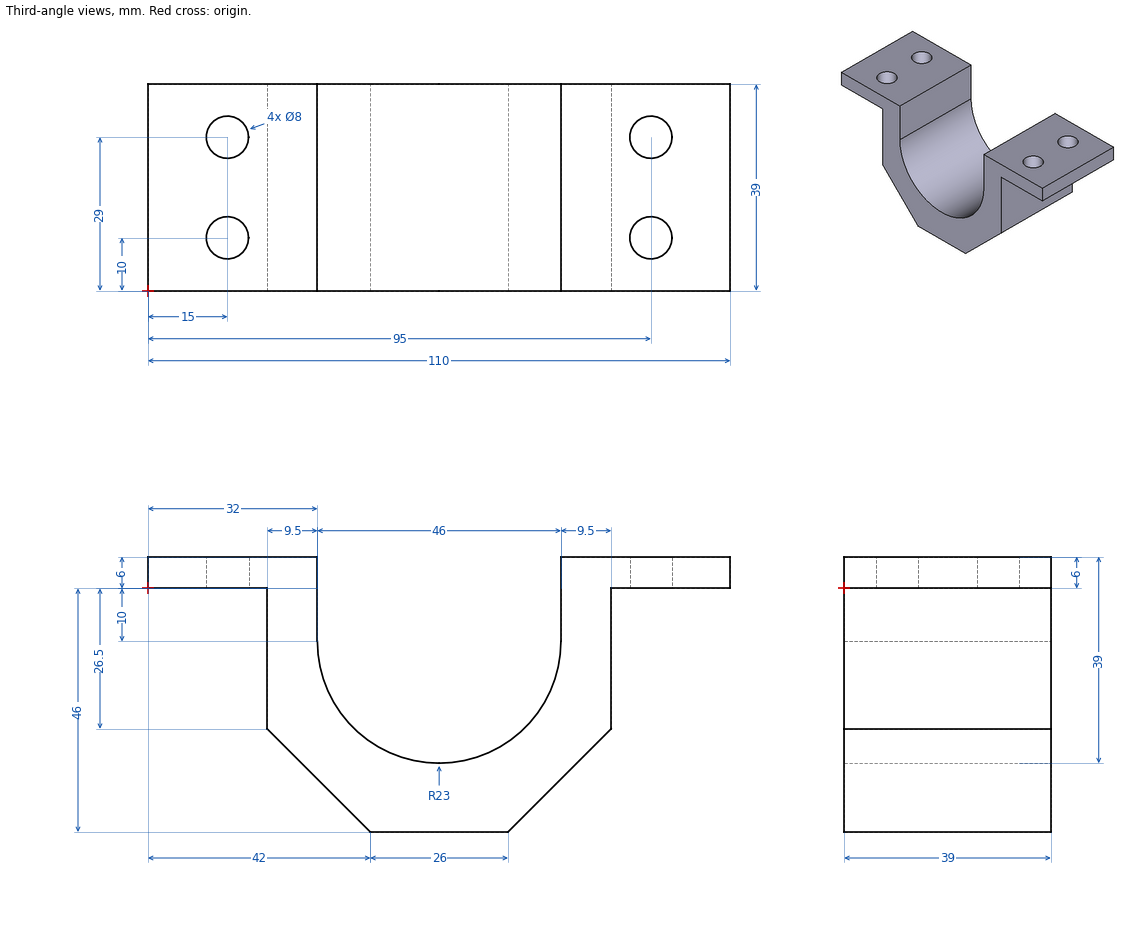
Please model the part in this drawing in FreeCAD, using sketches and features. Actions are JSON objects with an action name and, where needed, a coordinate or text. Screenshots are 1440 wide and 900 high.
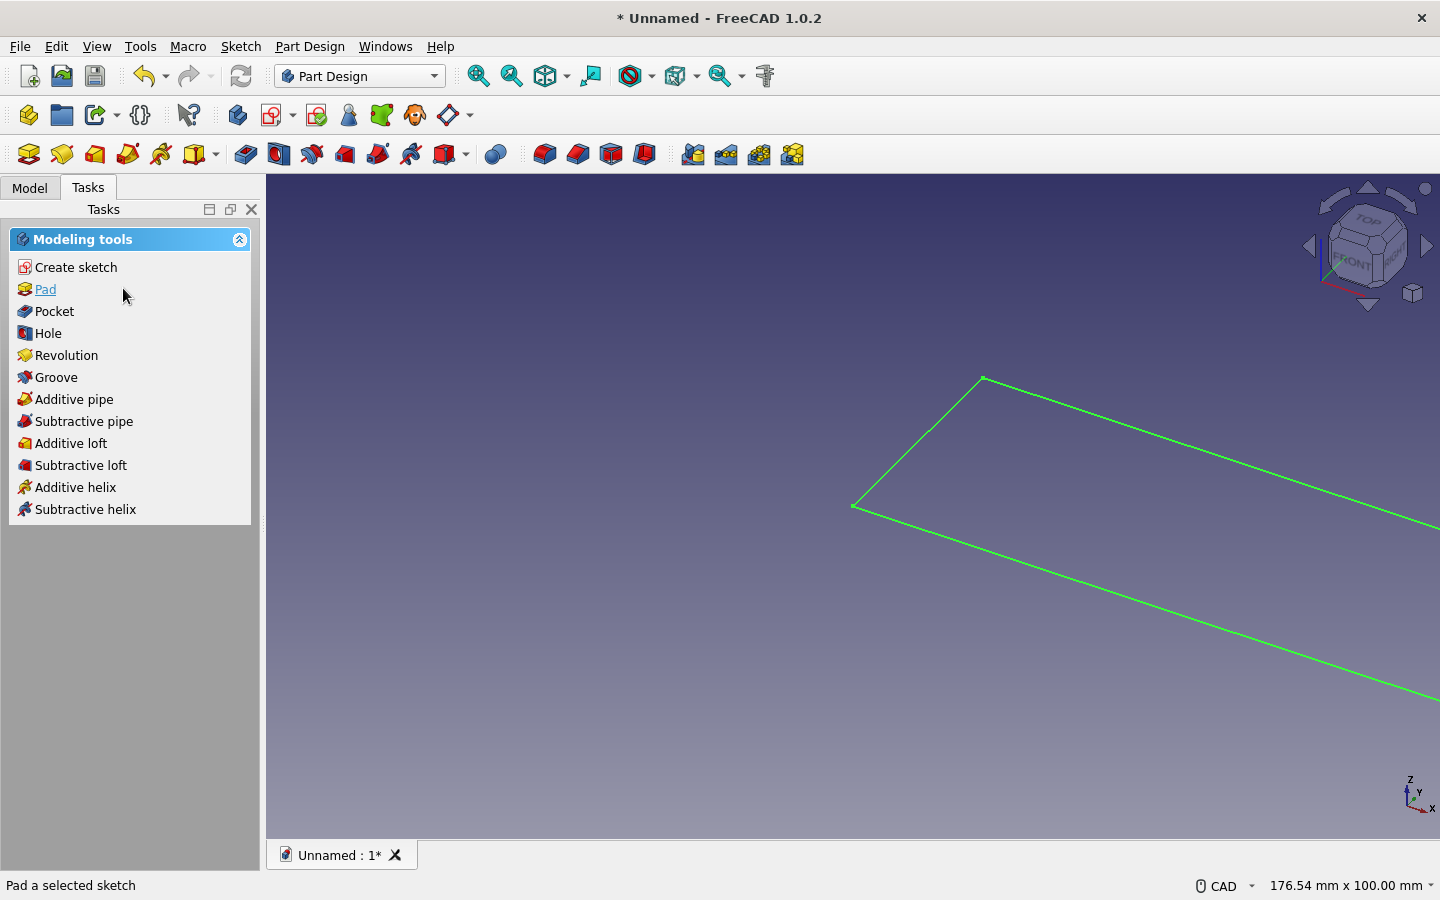
{"action": "left_click", "coordinate": [29, 154]}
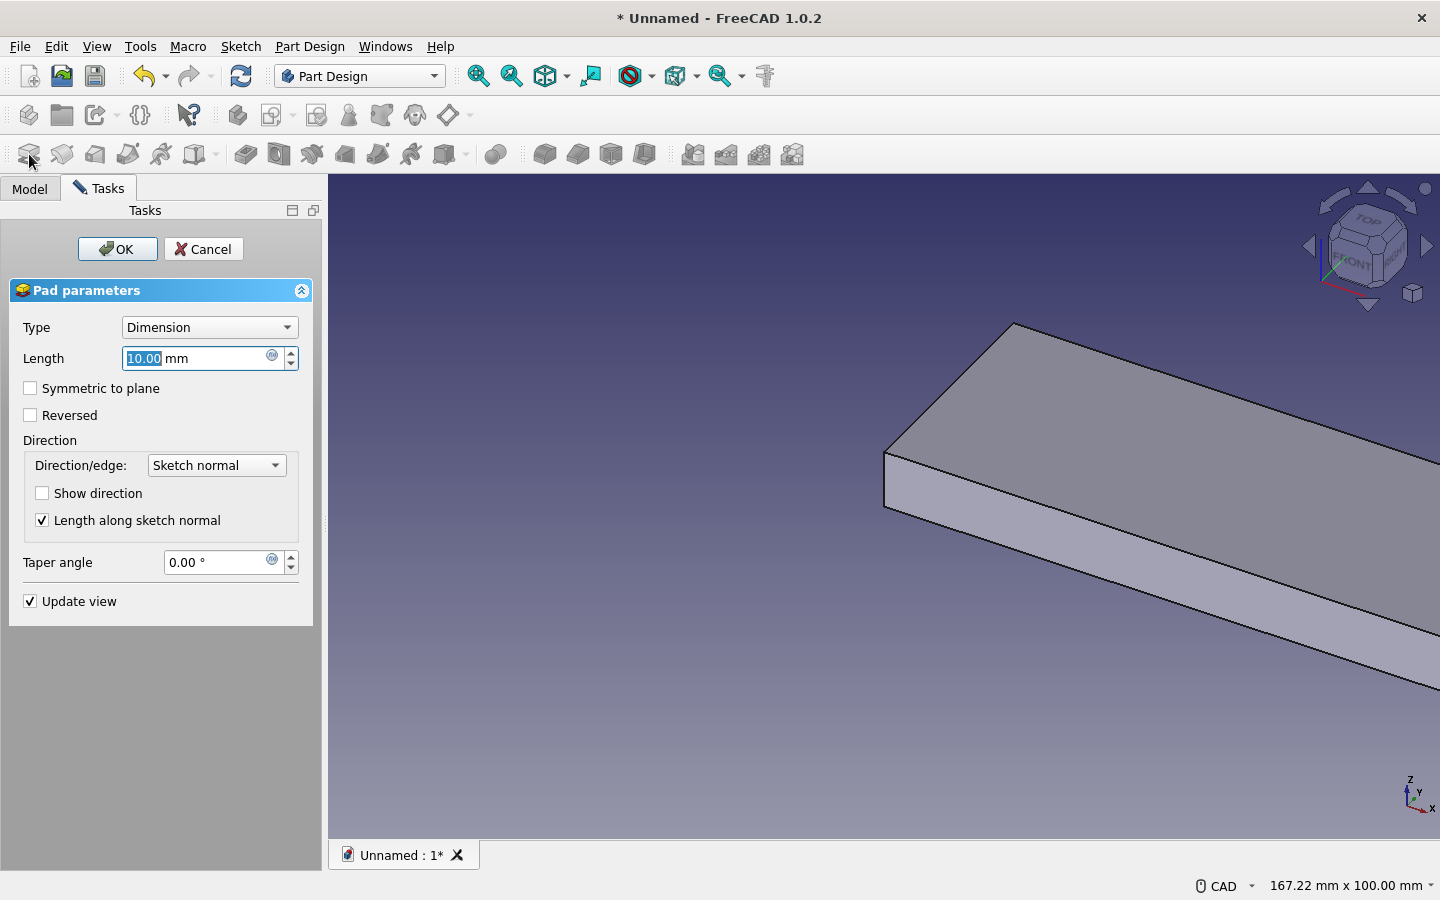
{"action": "type", "text": "6"}
{"action": "key", "text": "Tab"}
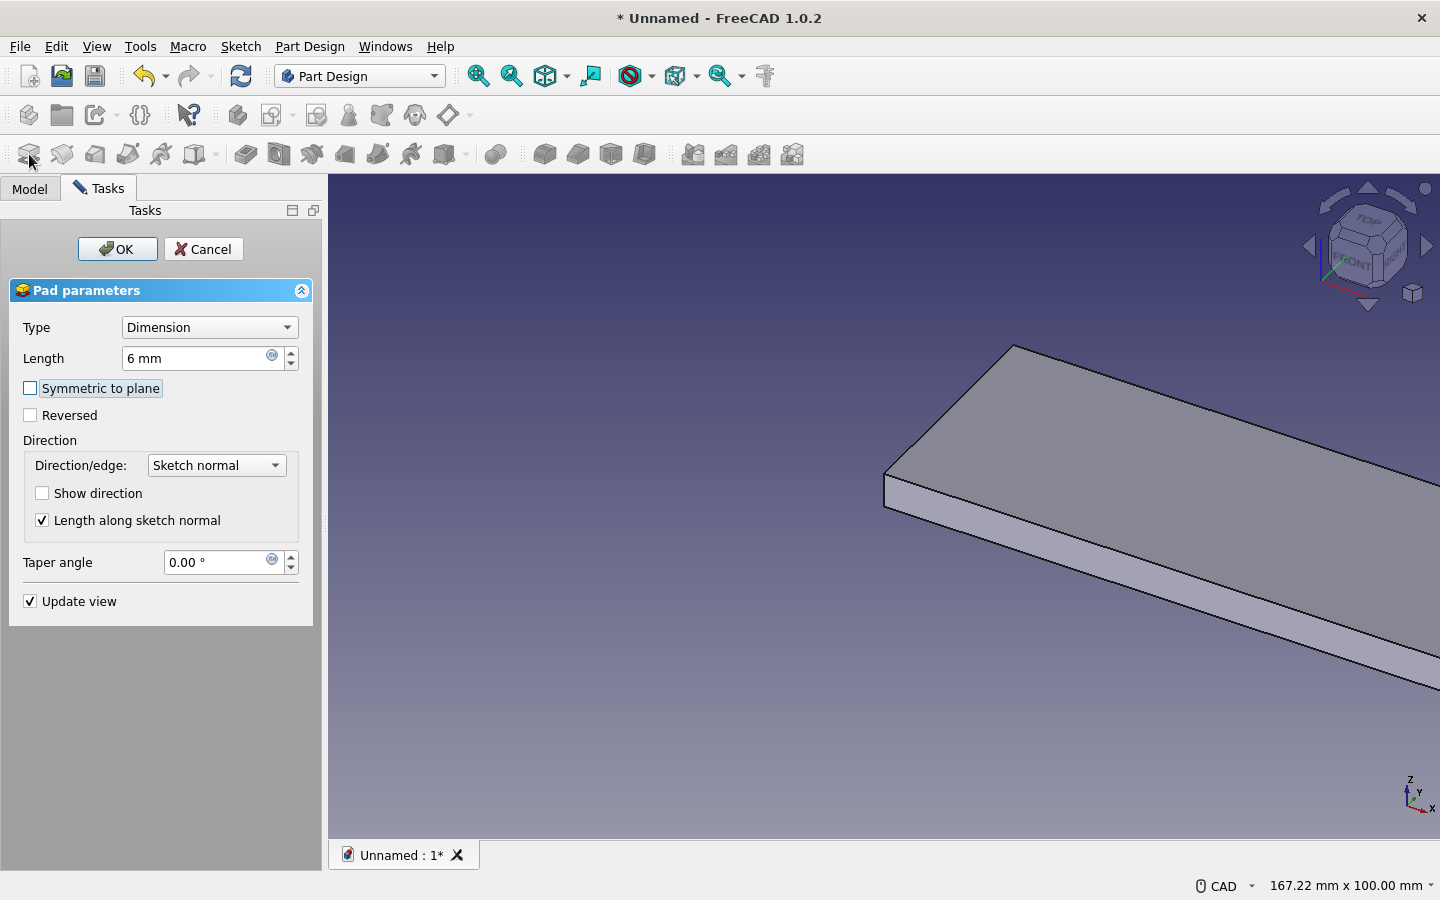
{"action": "left_click", "coordinate": [118, 249]}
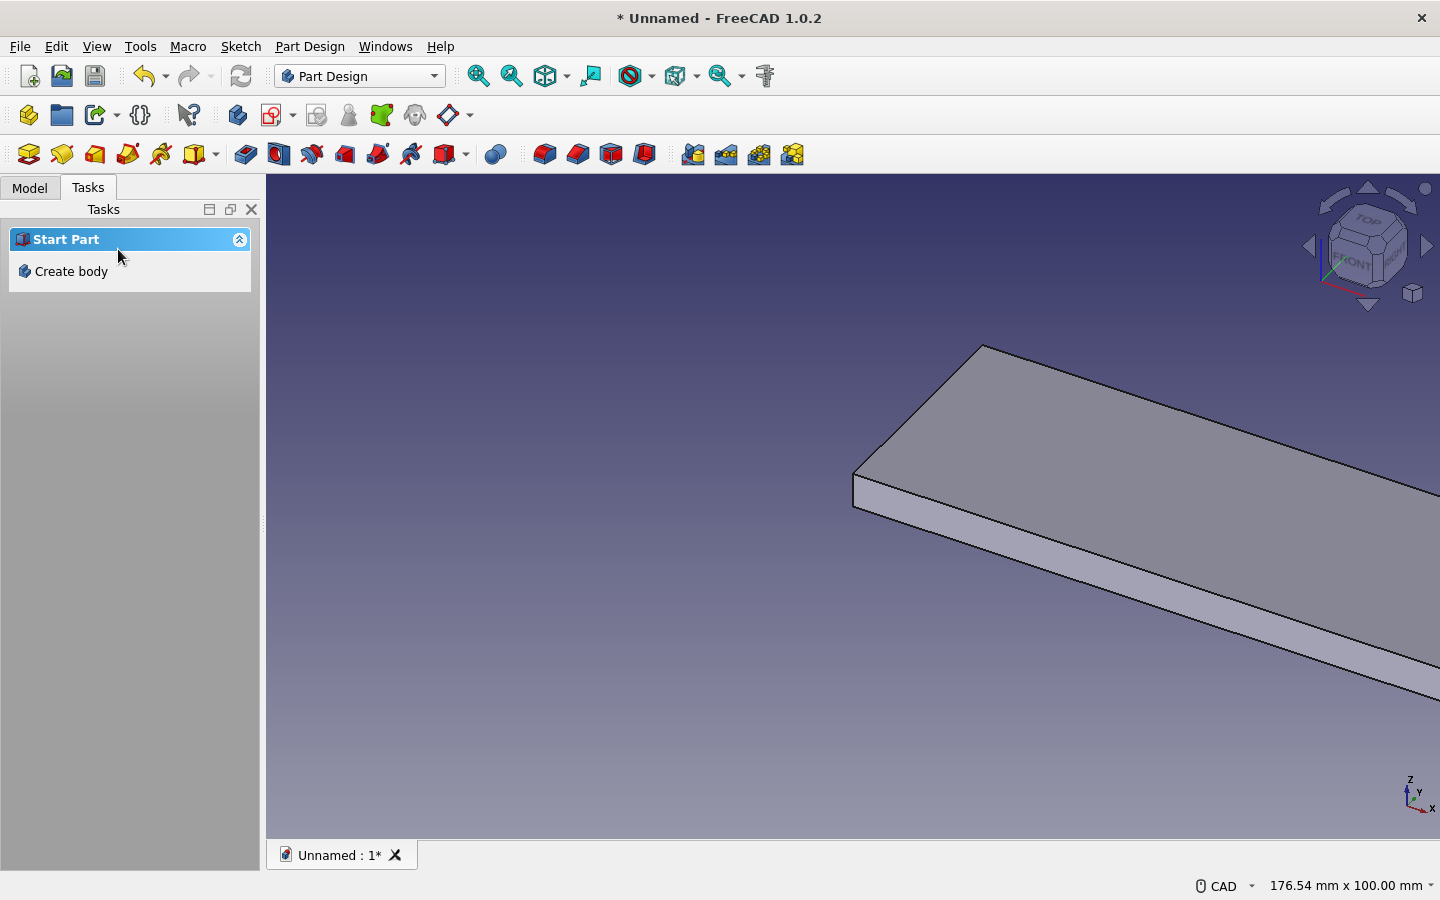
{"action": "key", "text": "v f"}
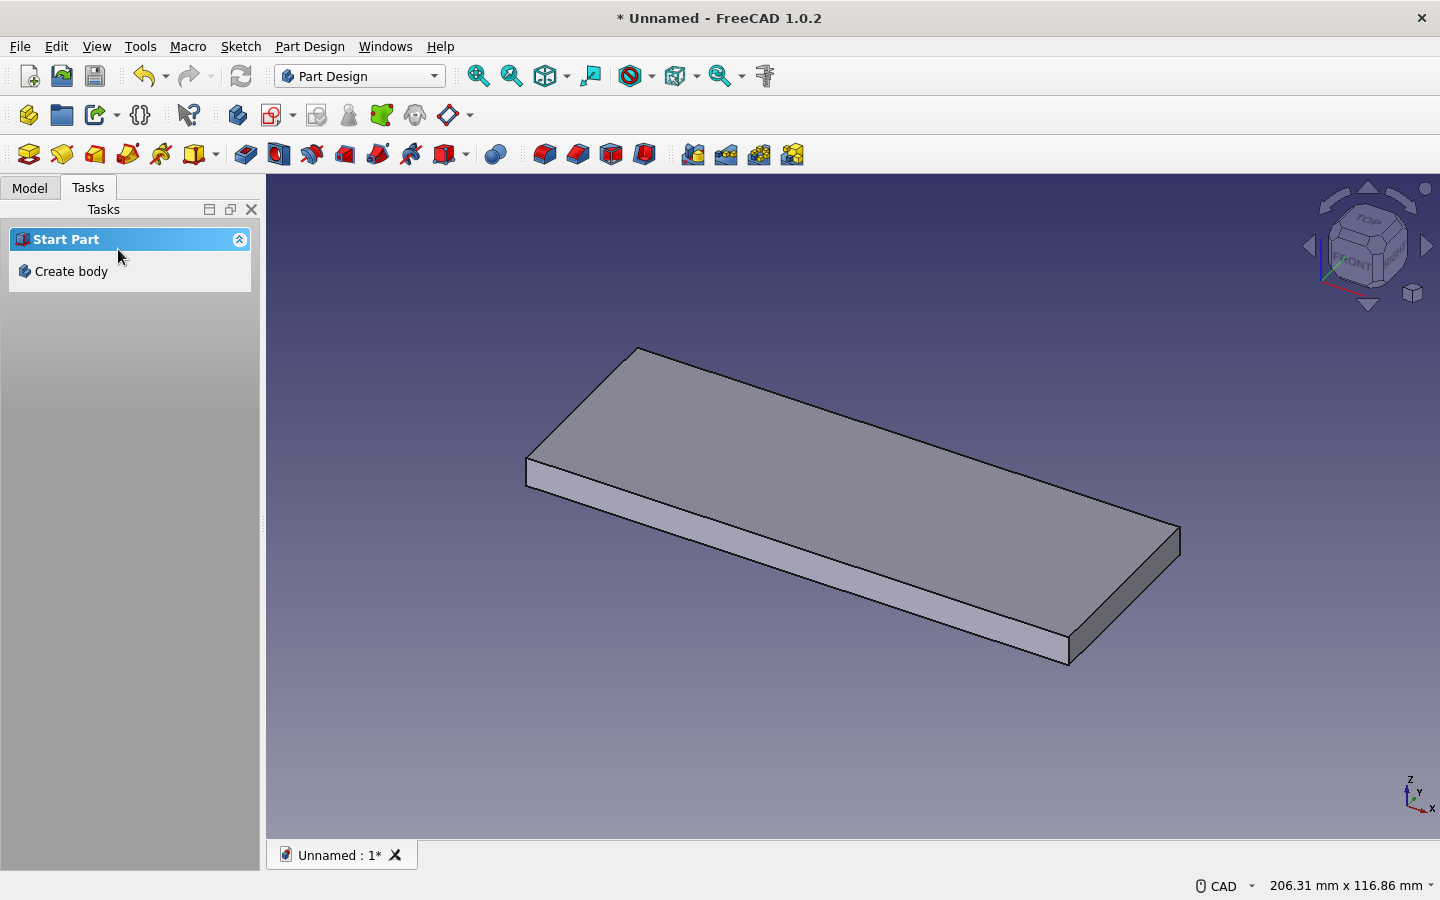
{"action": "left_click", "coordinate": [270, 116]}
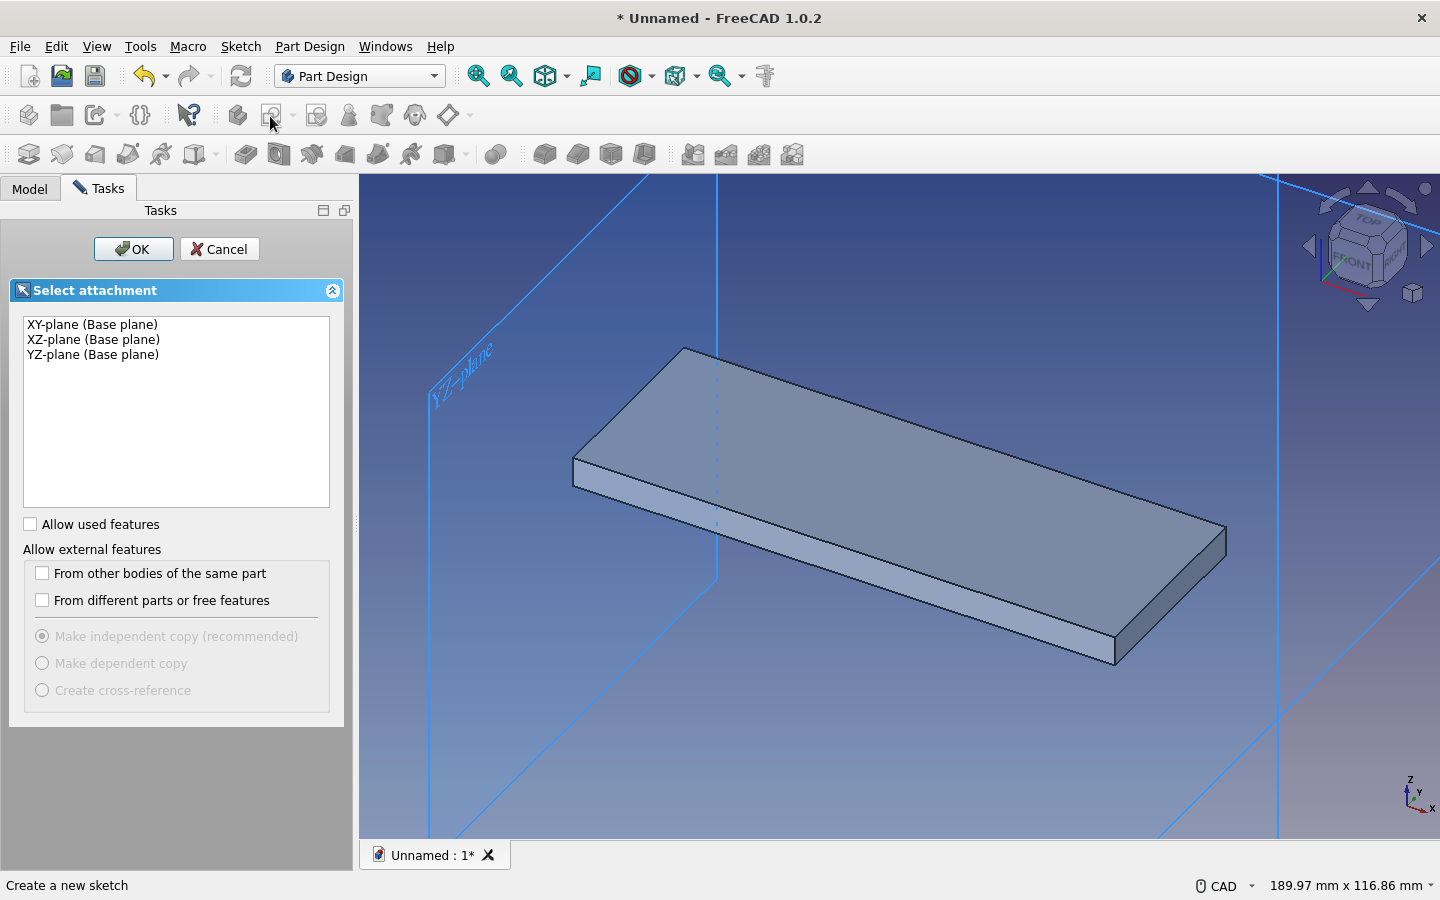
{"action": "left_click", "coordinate": [84, 340]}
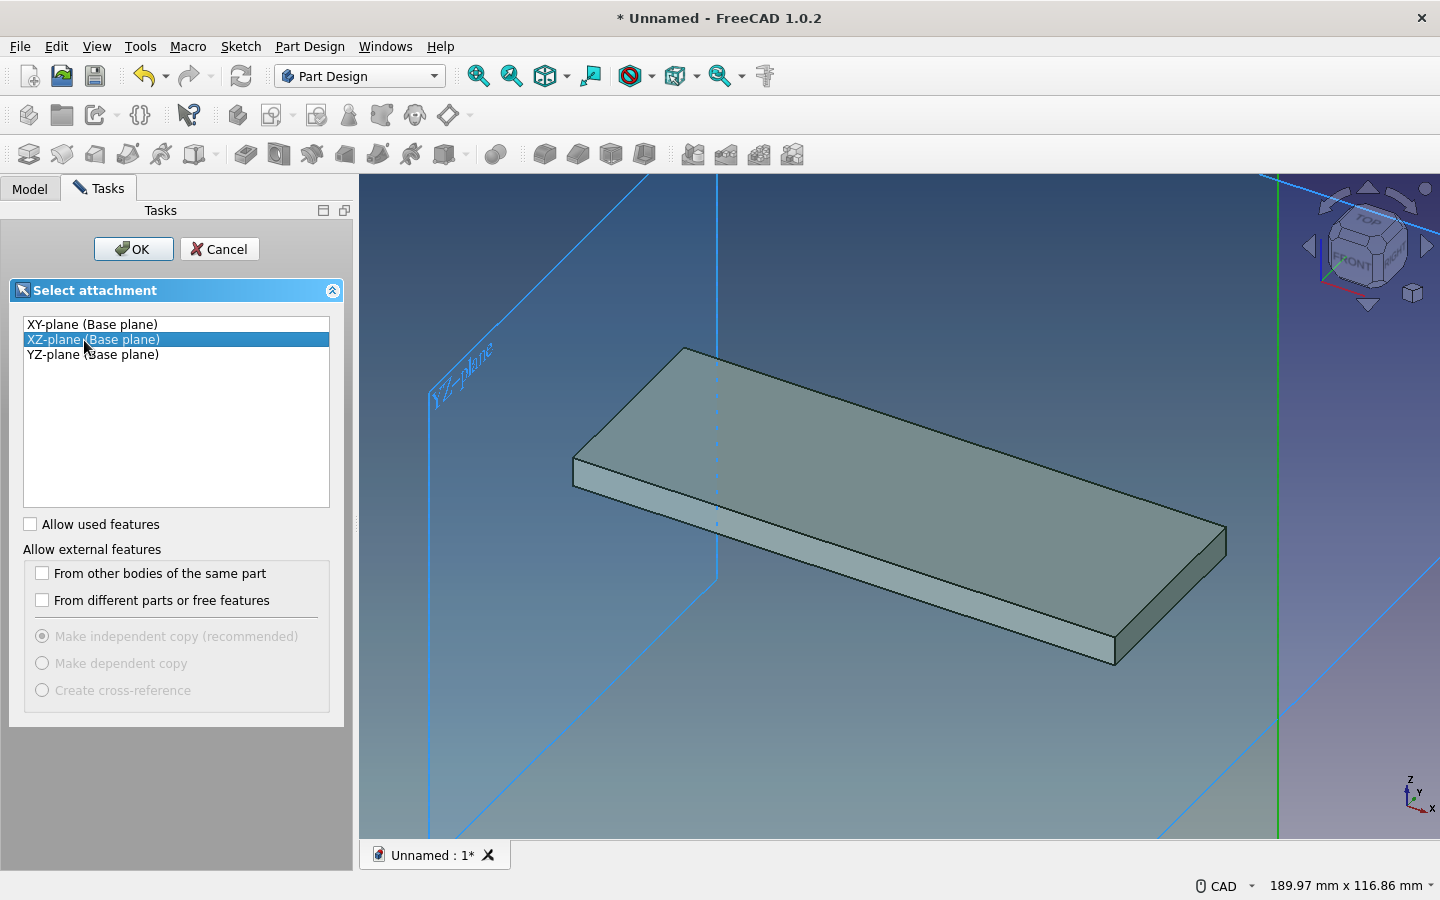
{"action": "left_click", "coordinate": [134, 249]}